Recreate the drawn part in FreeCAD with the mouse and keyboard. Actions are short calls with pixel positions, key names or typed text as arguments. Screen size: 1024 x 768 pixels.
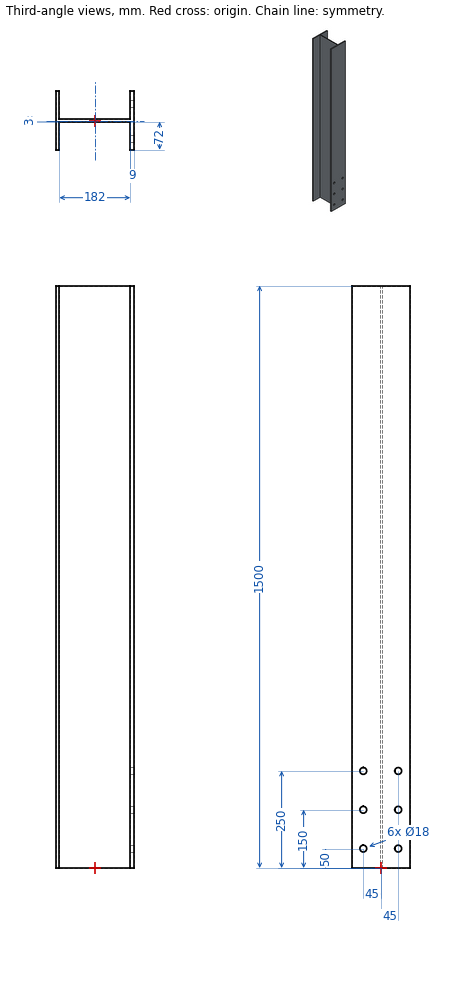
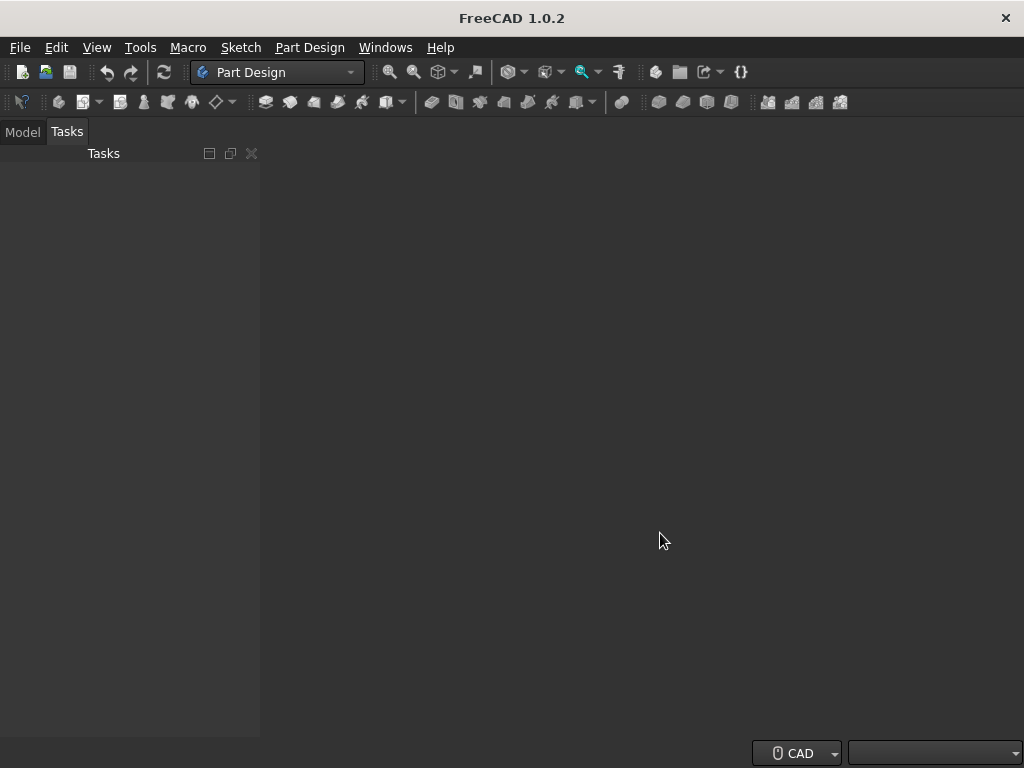
click(22, 72)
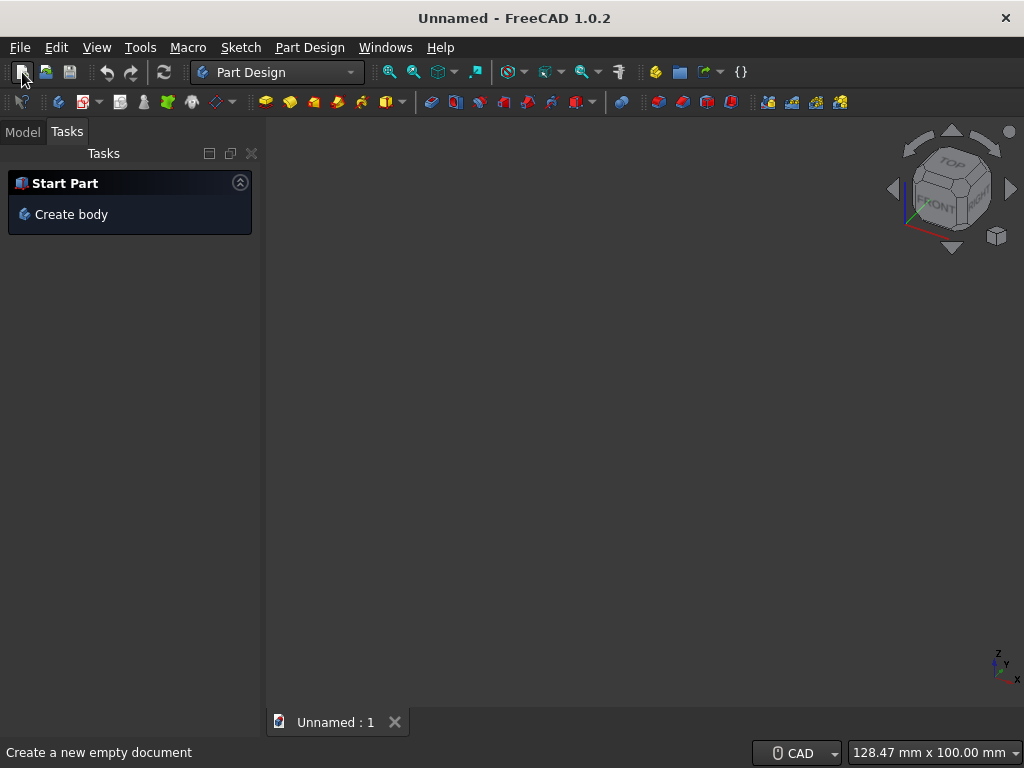
click(84, 102)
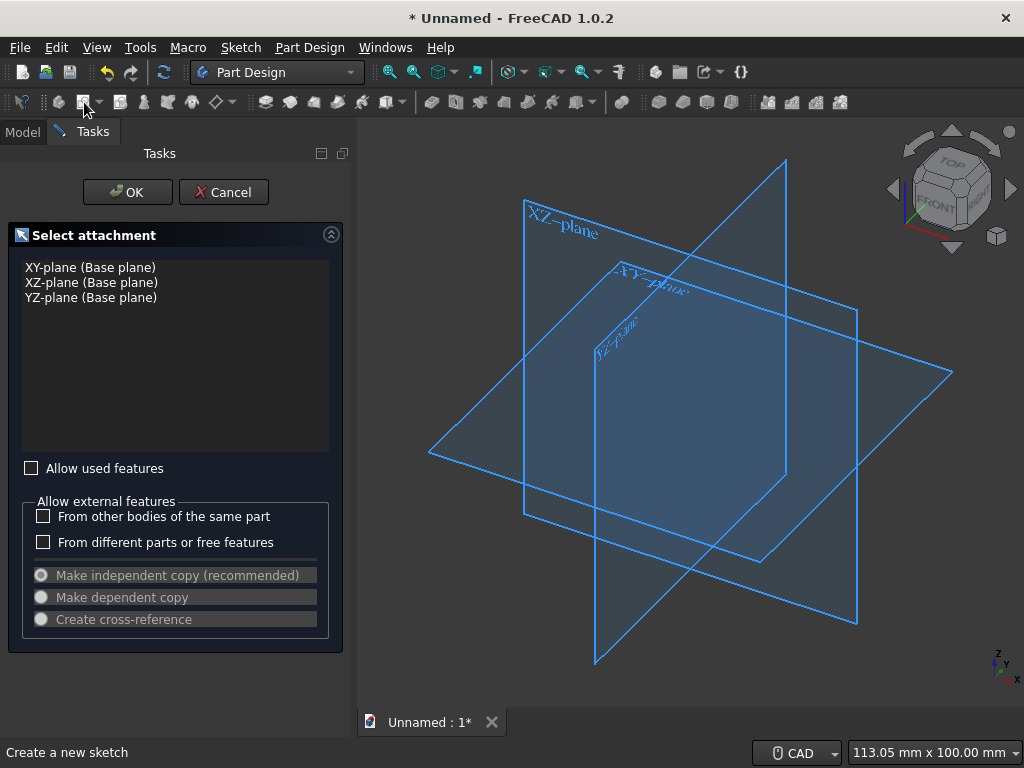
click(82, 268)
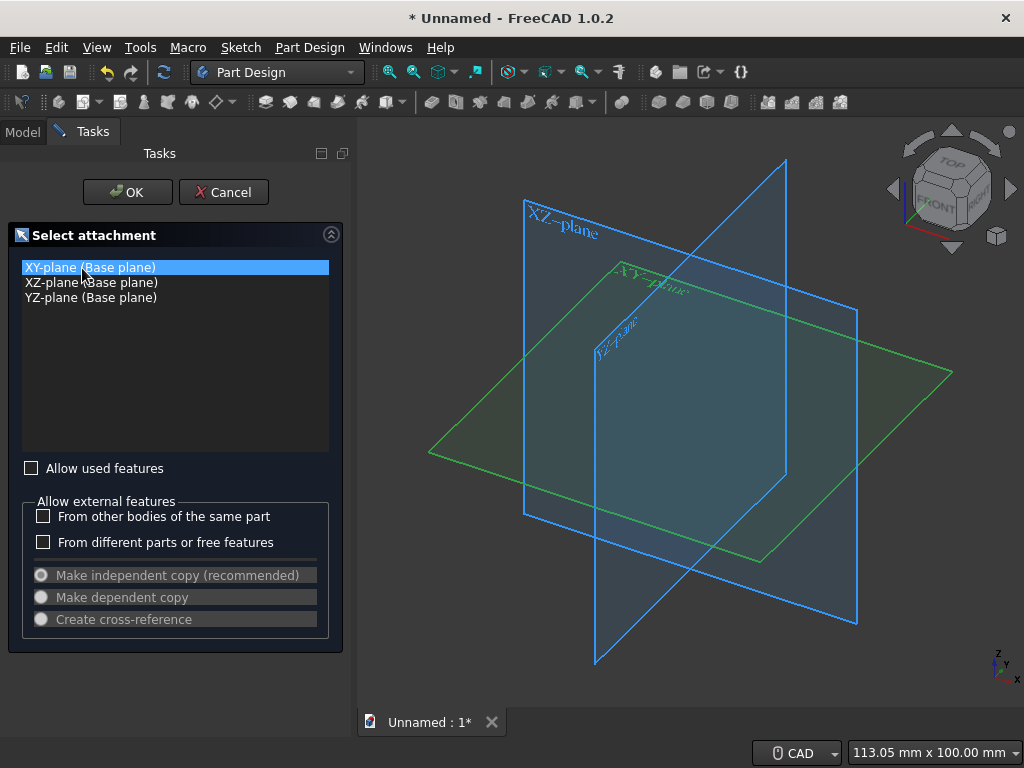
click(128, 192)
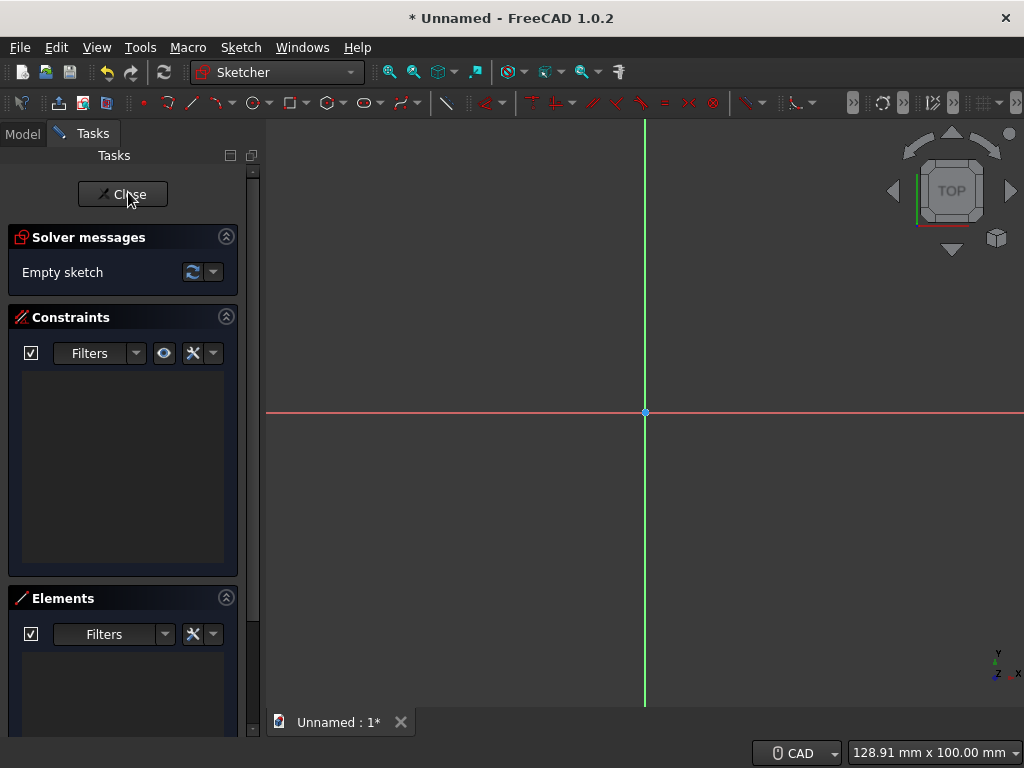
scroll(537, 413, down, 5)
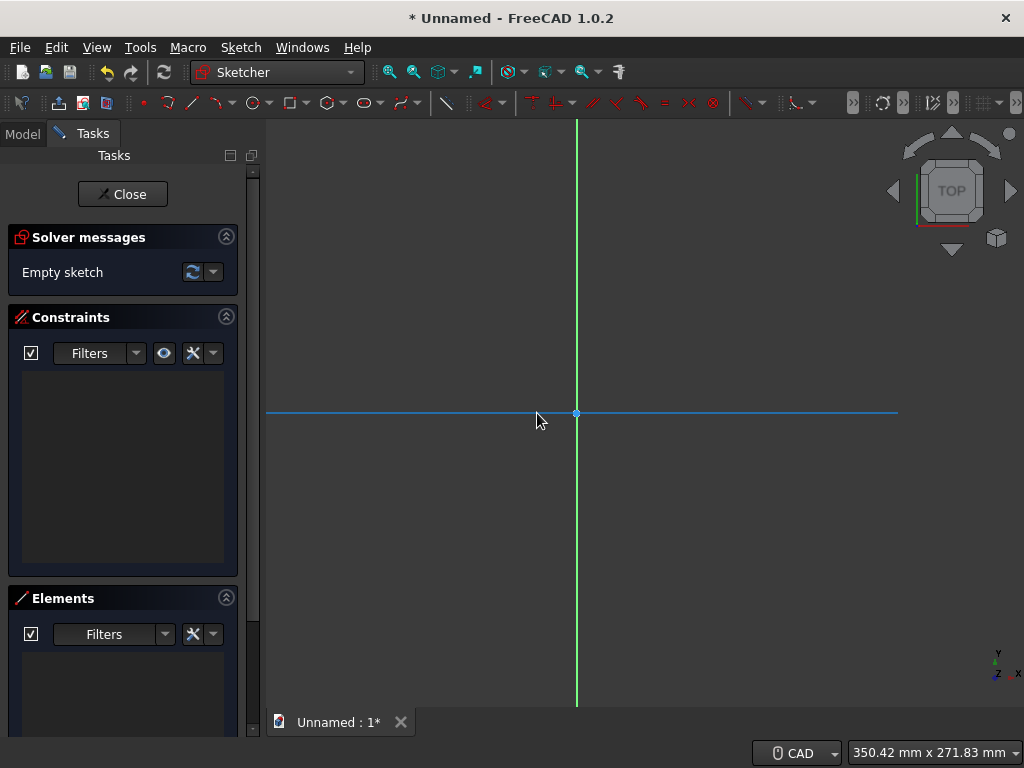
click(168, 104)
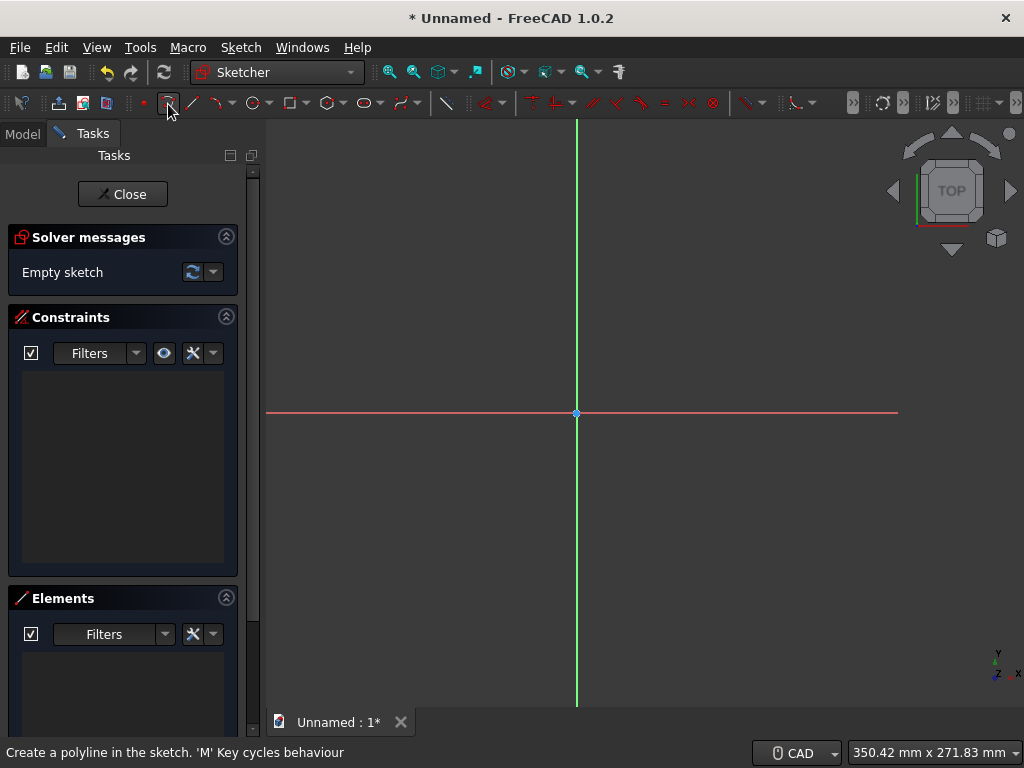
scroll(380, 420, up, 5)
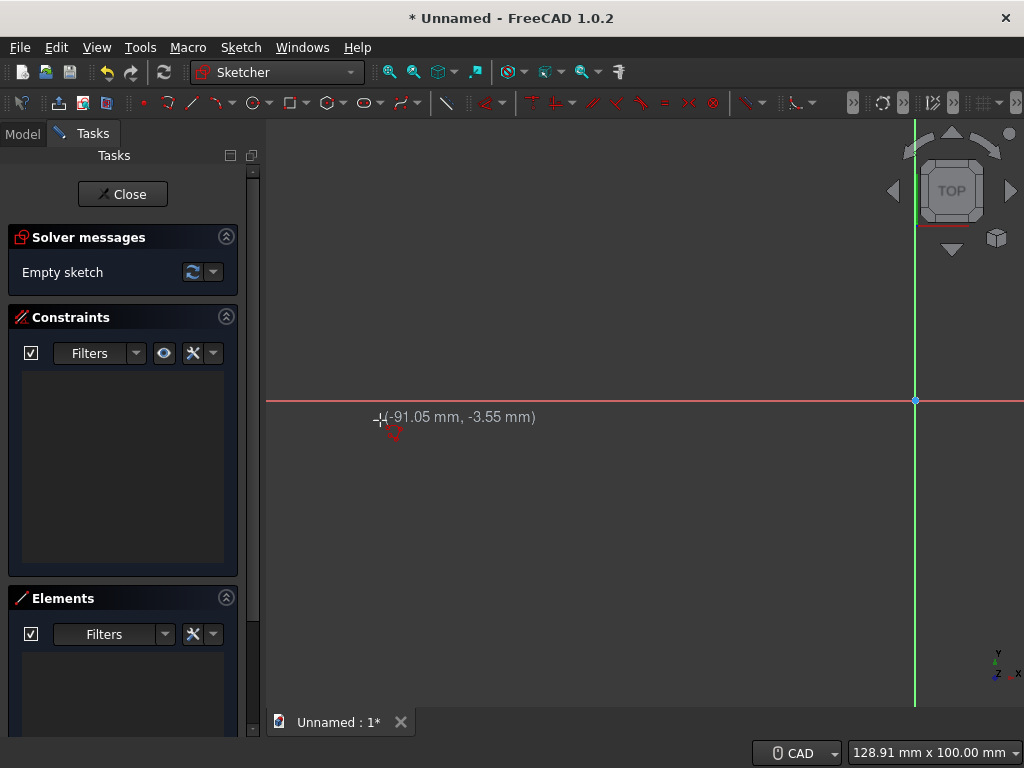
click(380, 419)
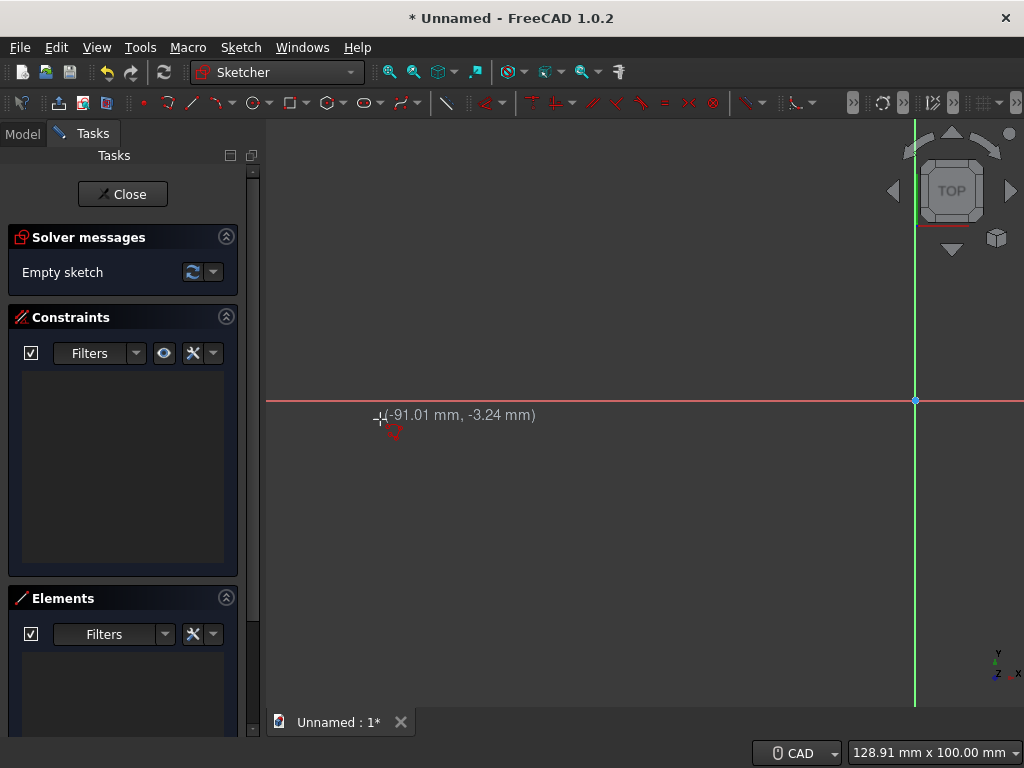
scroll(379, 420, down, 5)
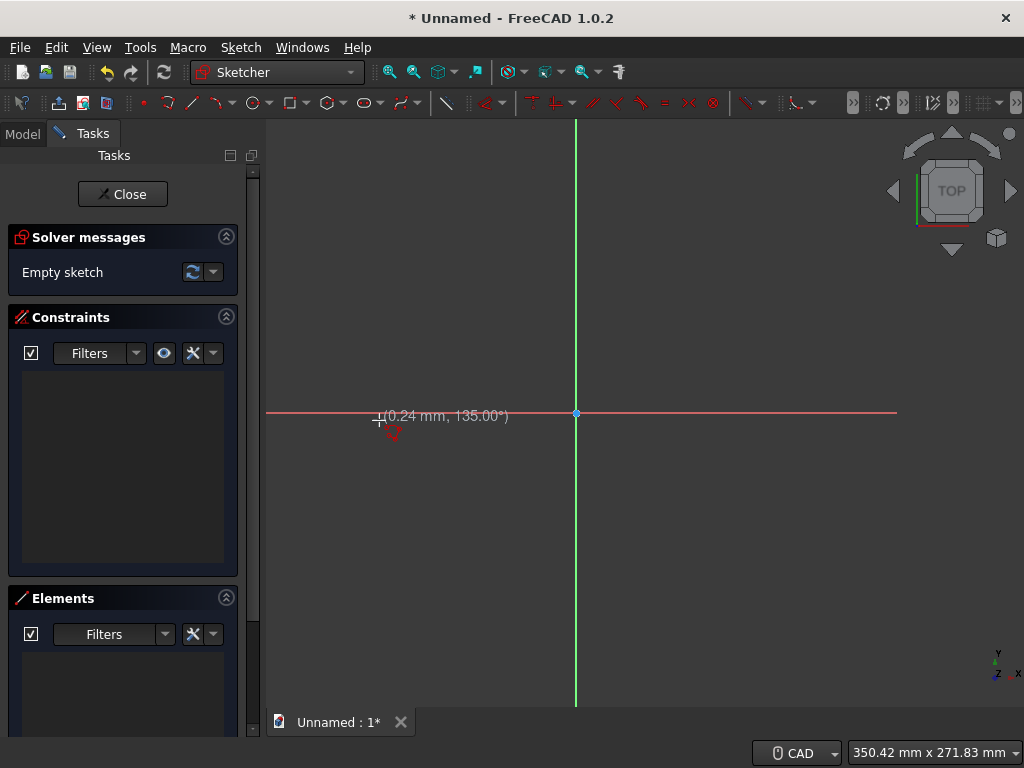
scroll(773, 420, up, 5)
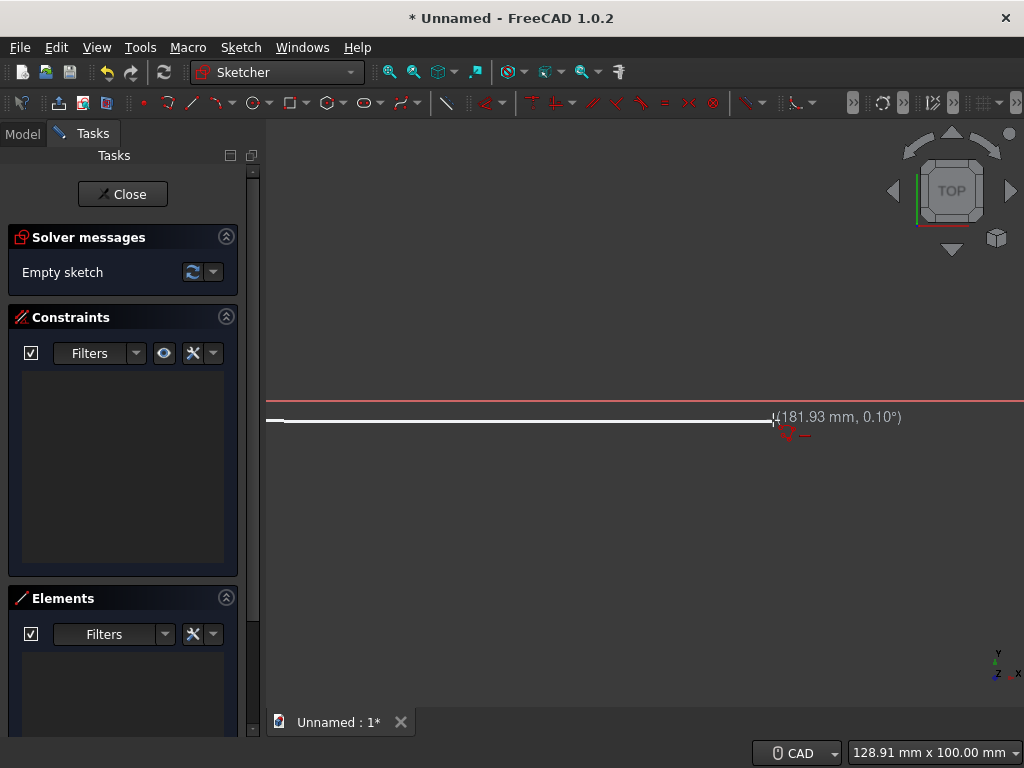
click(772, 419)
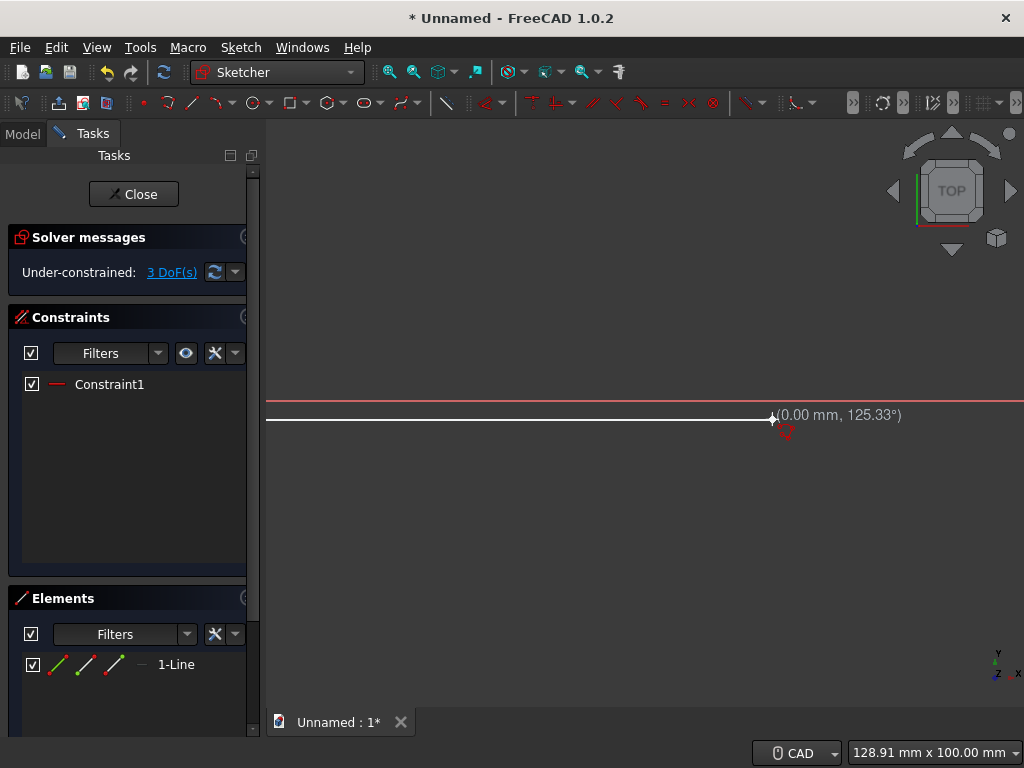
scroll(774, 420, down, 5)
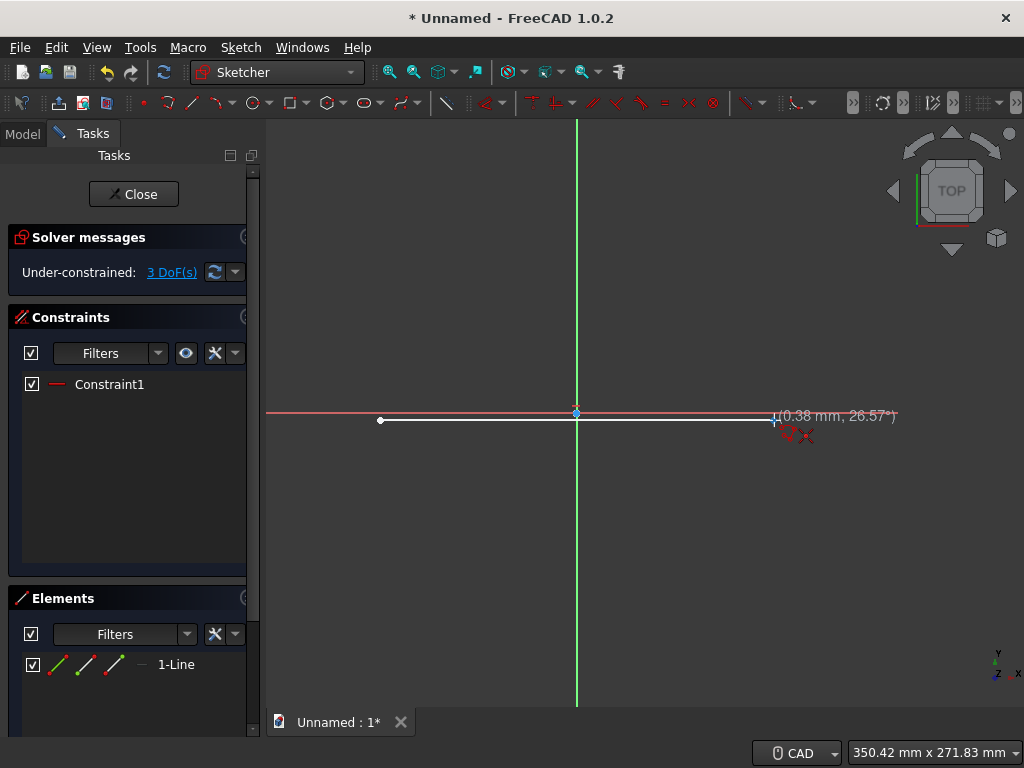
click(774, 576)
click(793, 576)
click(793, 251)
click(774, 251)